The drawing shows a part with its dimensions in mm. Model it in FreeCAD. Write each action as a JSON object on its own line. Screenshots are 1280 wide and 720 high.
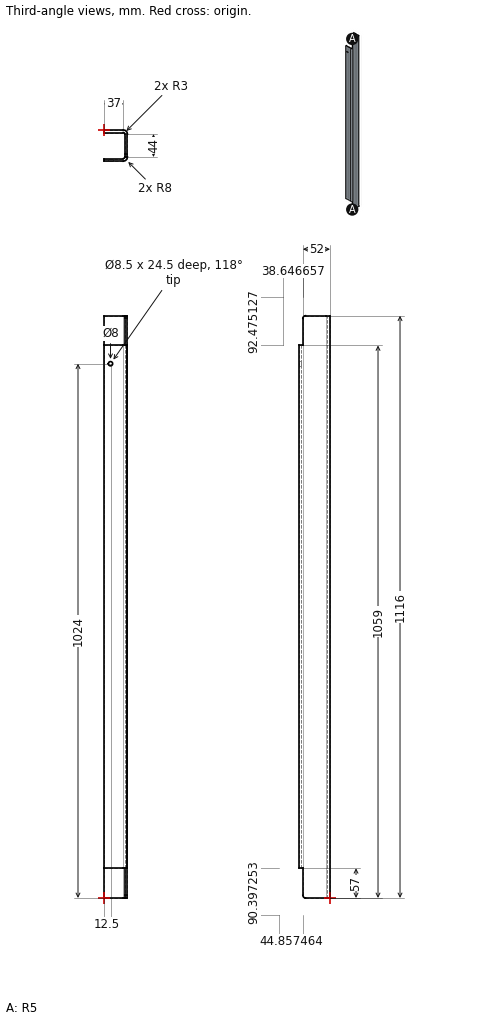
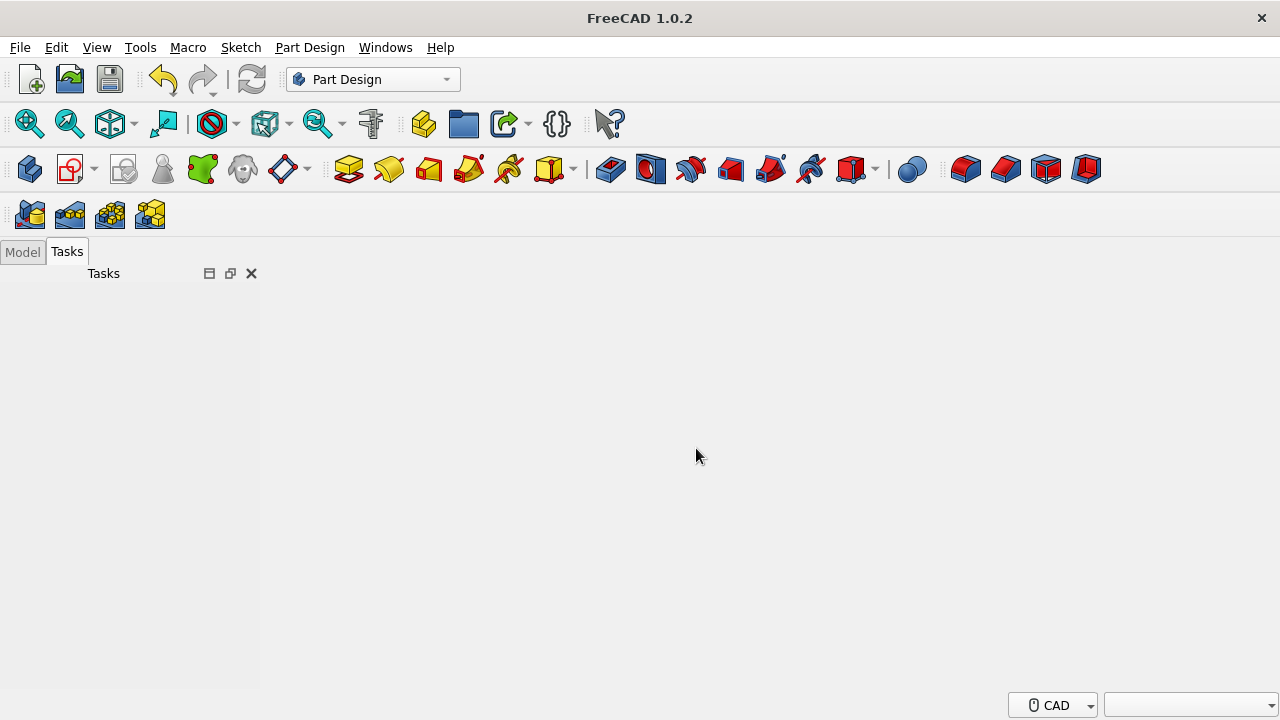
{"action": "key", "text": "ctrl+n"}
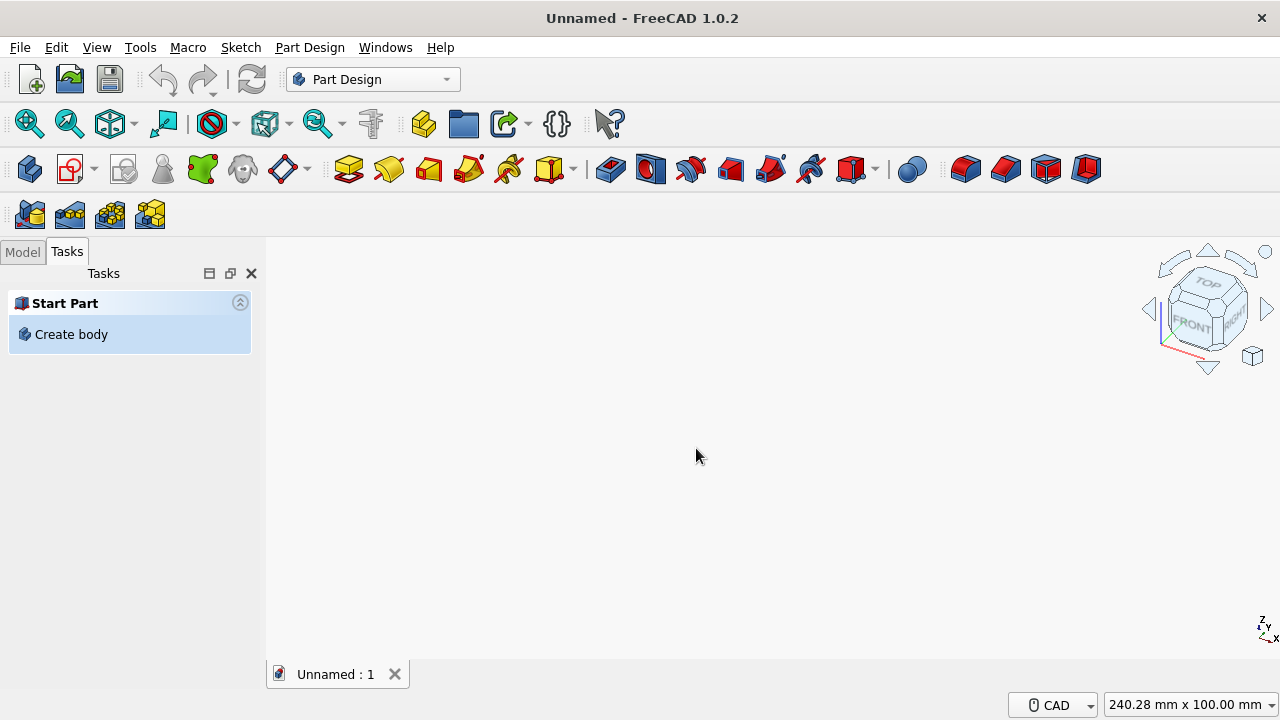
{"action": "left_click", "coordinate": [70, 170]}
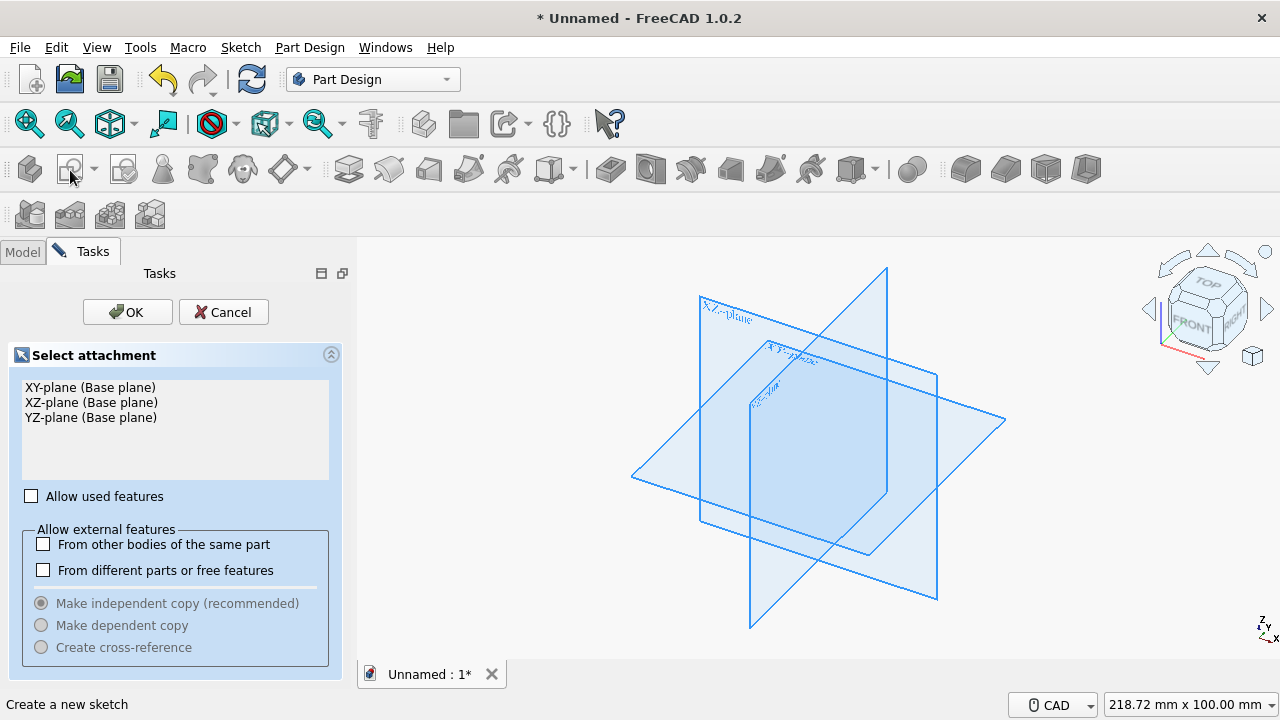
{"action": "left_click", "coordinate": [82, 388]}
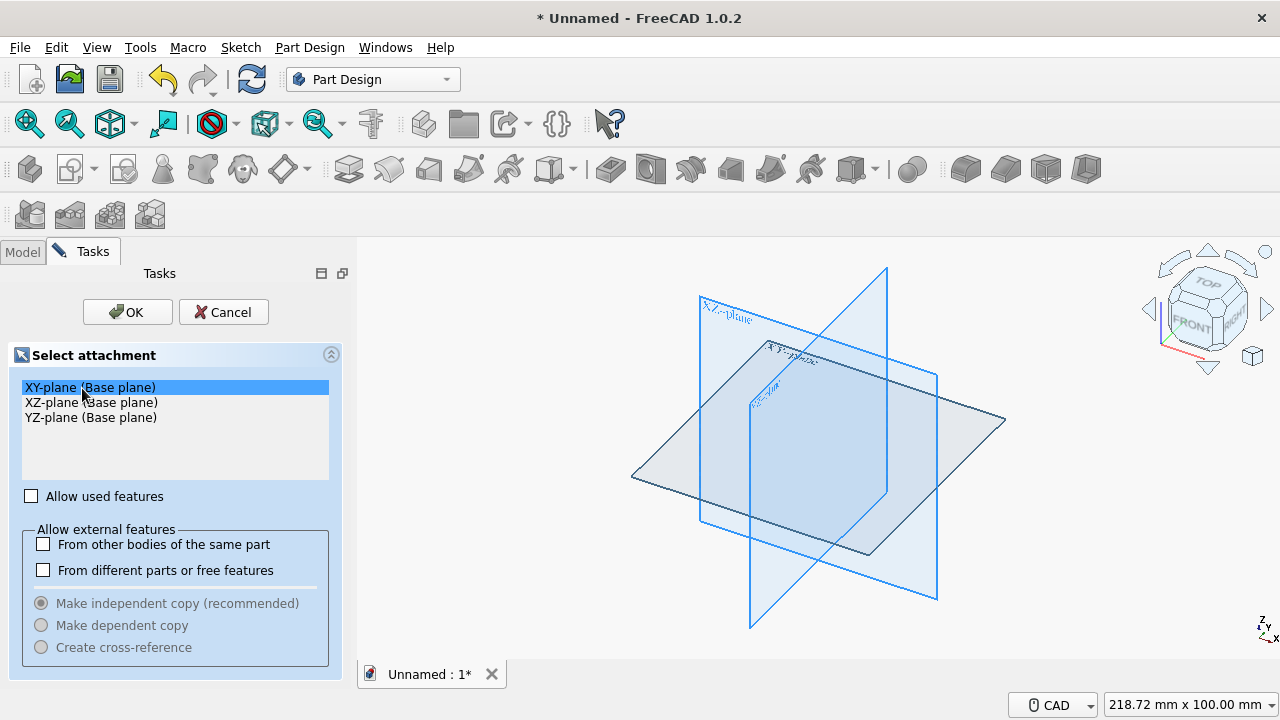
{"action": "left_click", "coordinate": [128, 312]}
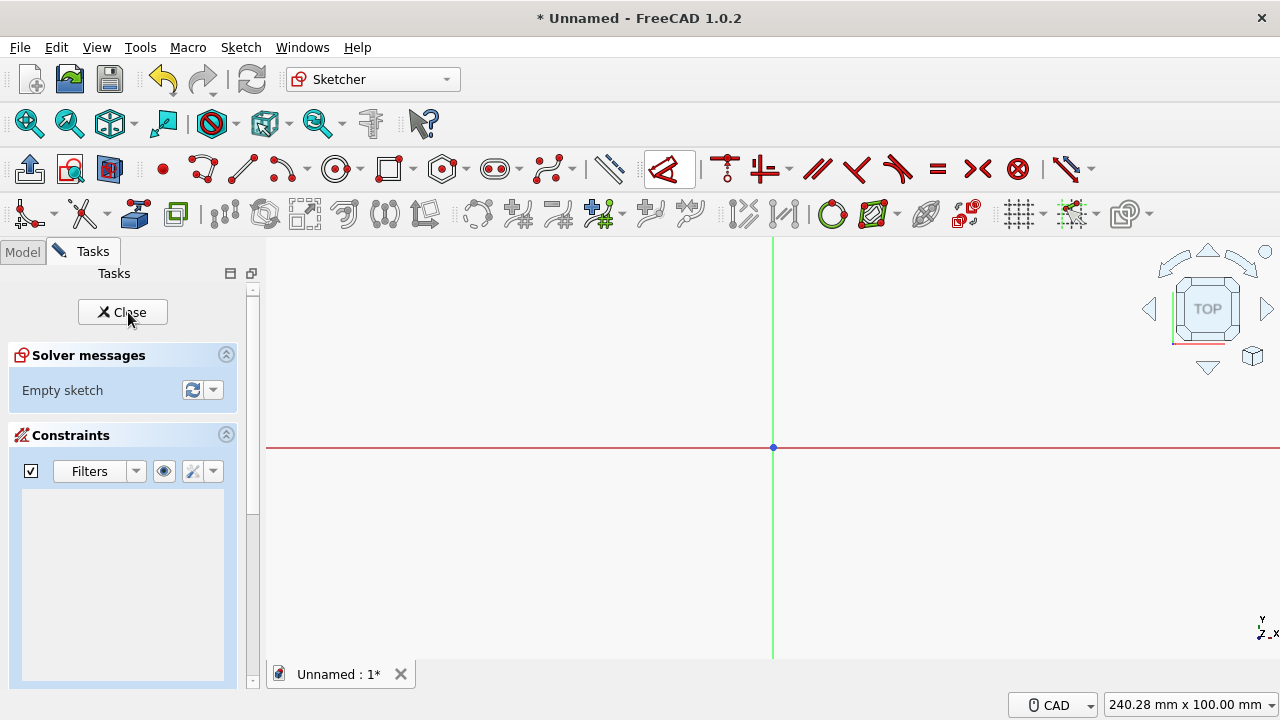
{"action": "scroll", "coordinate": [372, 265], "scroll_direction": "down", "scroll_amount": 2}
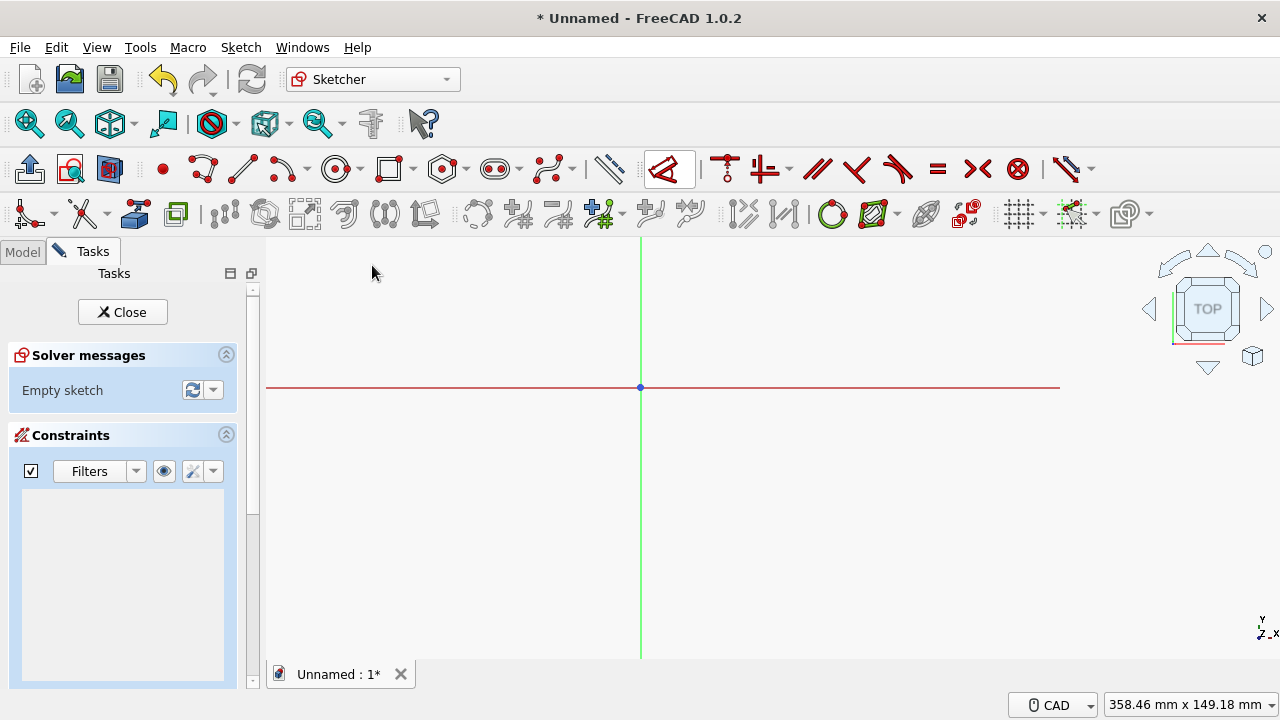
{"action": "scroll", "coordinate": [704, 522], "scroll_direction": "up", "scroll_amount": 2}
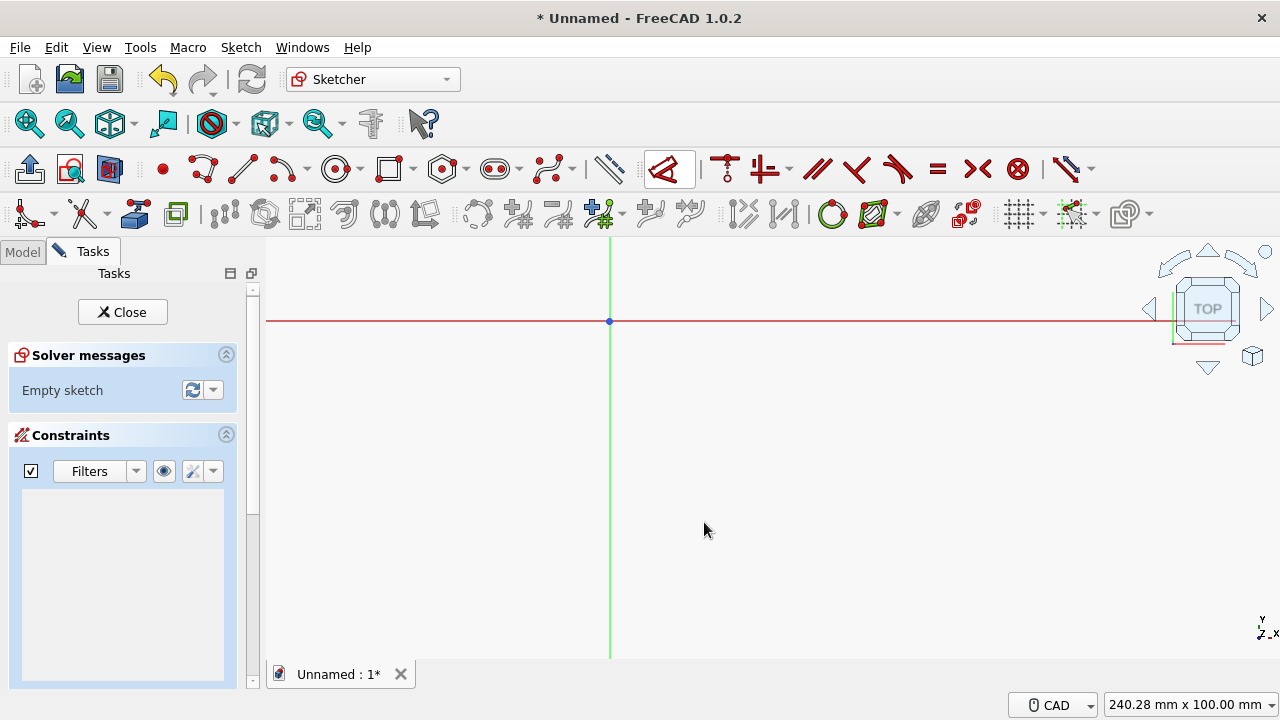
{"action": "key", "text": "g m"}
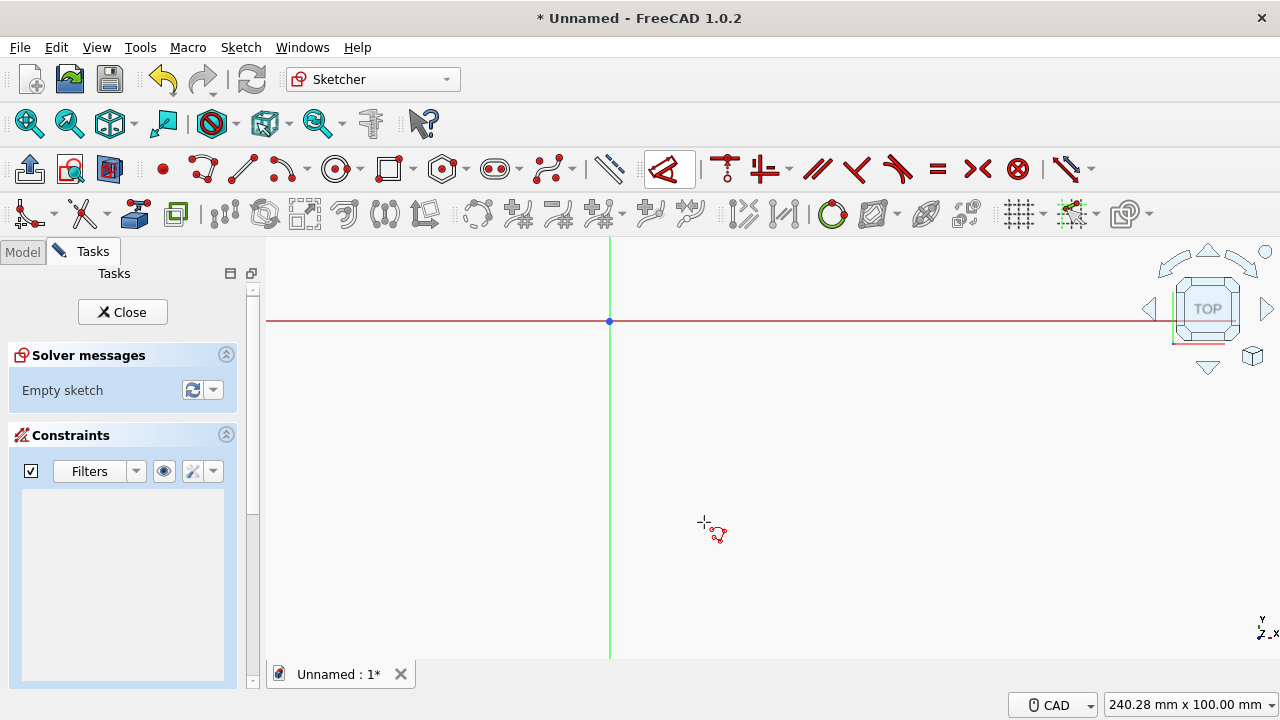
{"action": "left_click", "coordinate": [766, 321]}
{"action": "left_click", "coordinate": [610, 321]}
{"action": "left_click", "coordinate": [619, 342]}
{"action": "left_click", "coordinate": [766, 342]}
{"action": "right_click", "coordinate": [766, 342]}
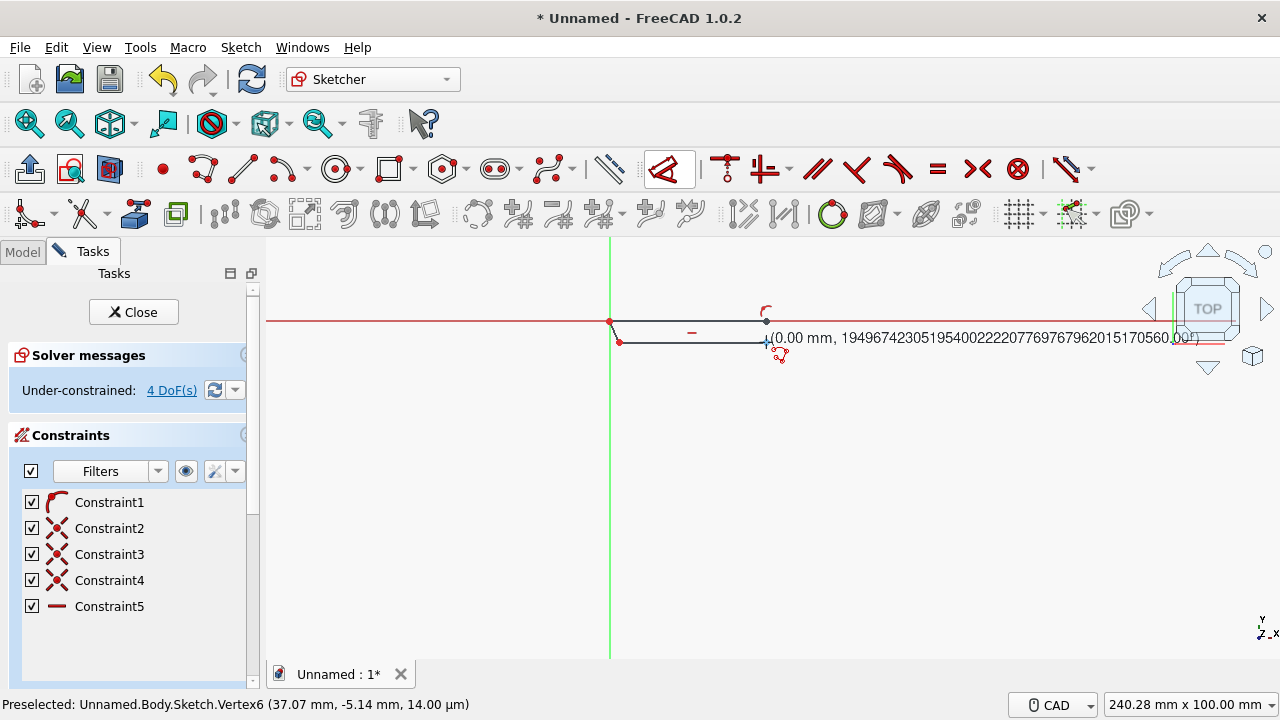
{"action": "left_click", "coordinate": [244, 170]}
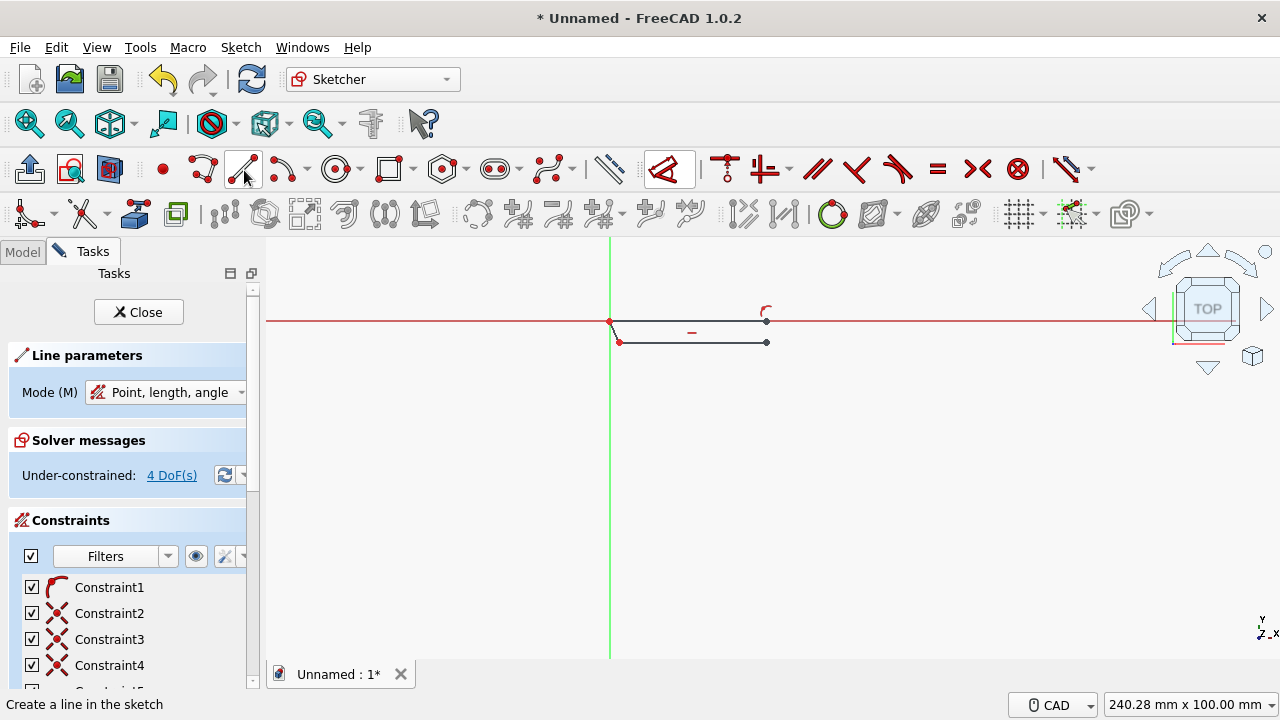
{"action": "left_click", "coordinate": [778, 355]}
{"action": "left_click", "coordinate": [778, 541]}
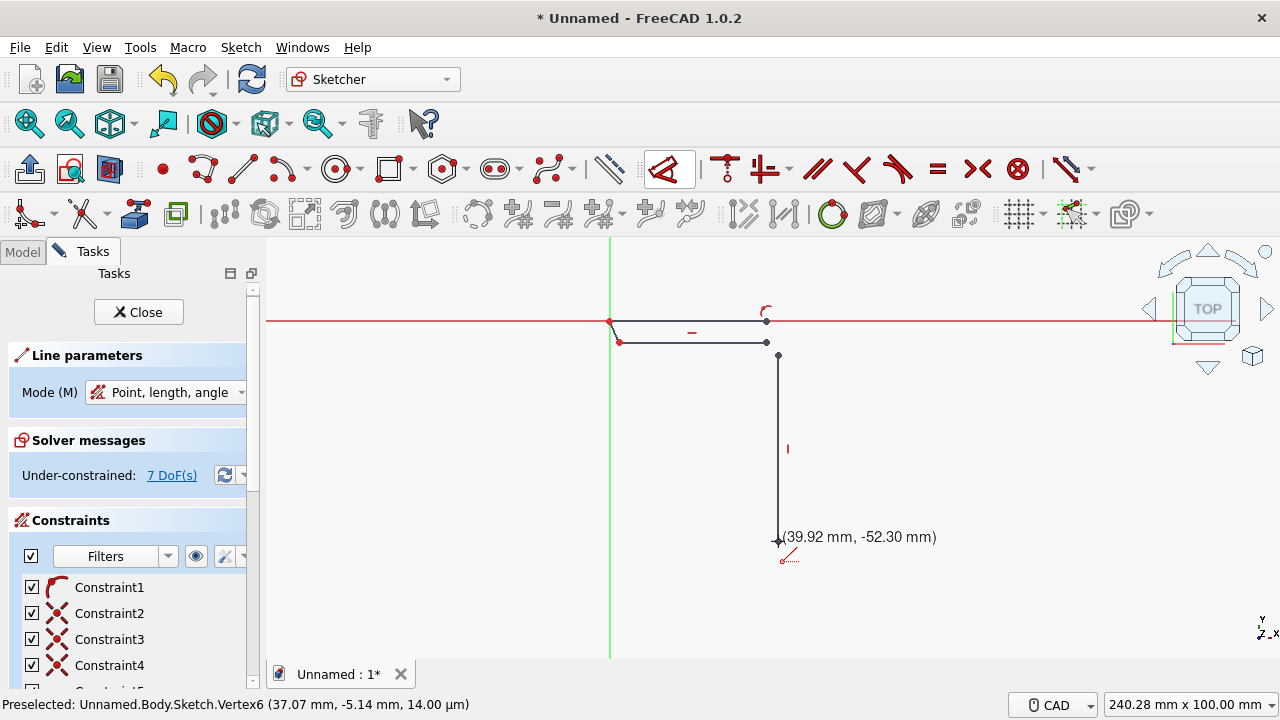
{"action": "key", "text": "g m"}